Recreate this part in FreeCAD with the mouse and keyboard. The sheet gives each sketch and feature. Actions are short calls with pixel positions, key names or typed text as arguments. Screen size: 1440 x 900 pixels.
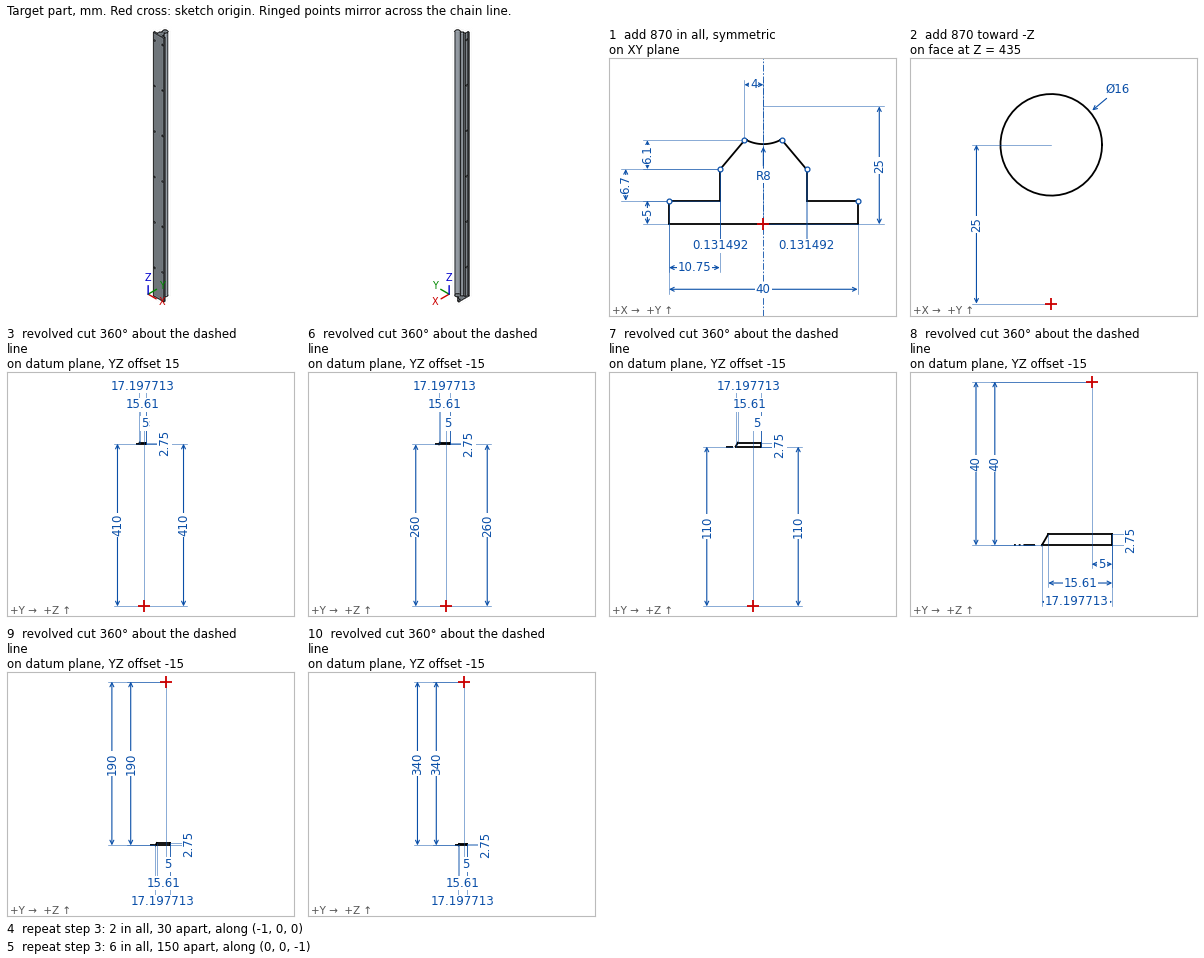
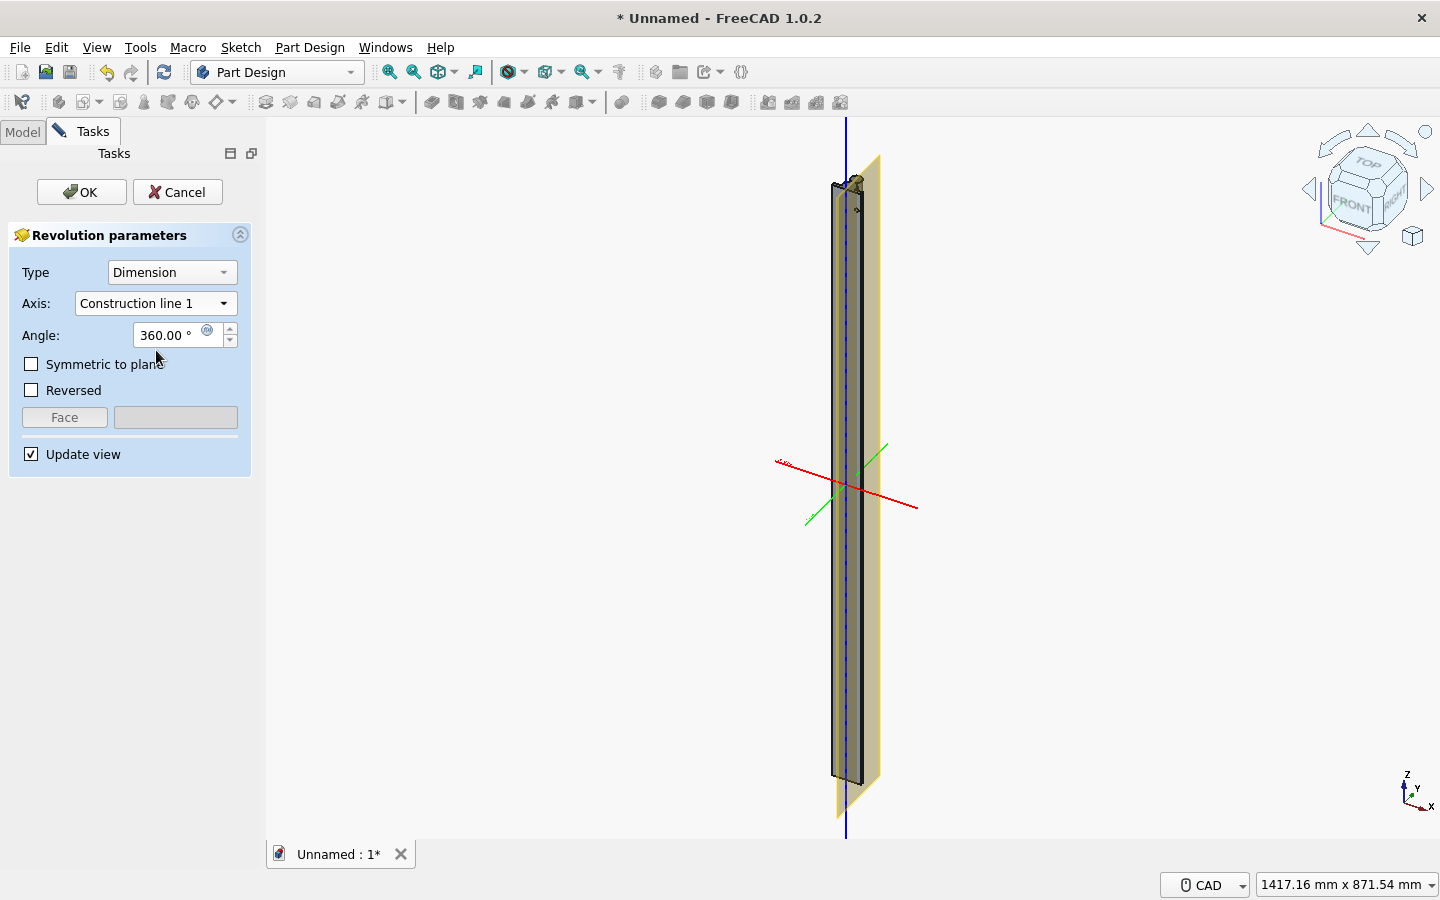
click(82, 192)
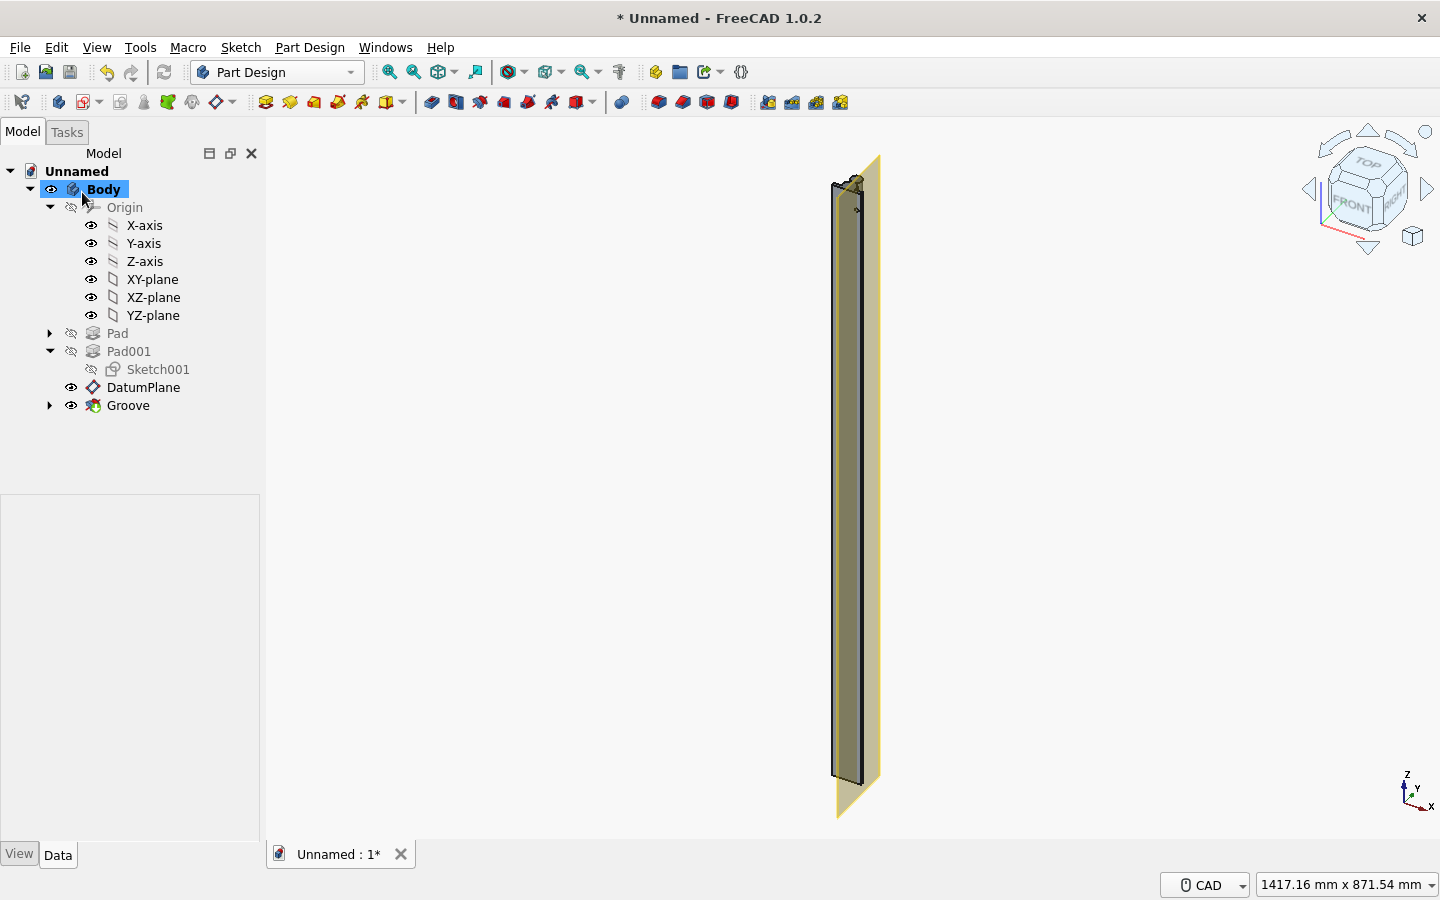
click(116, 387)
key(space)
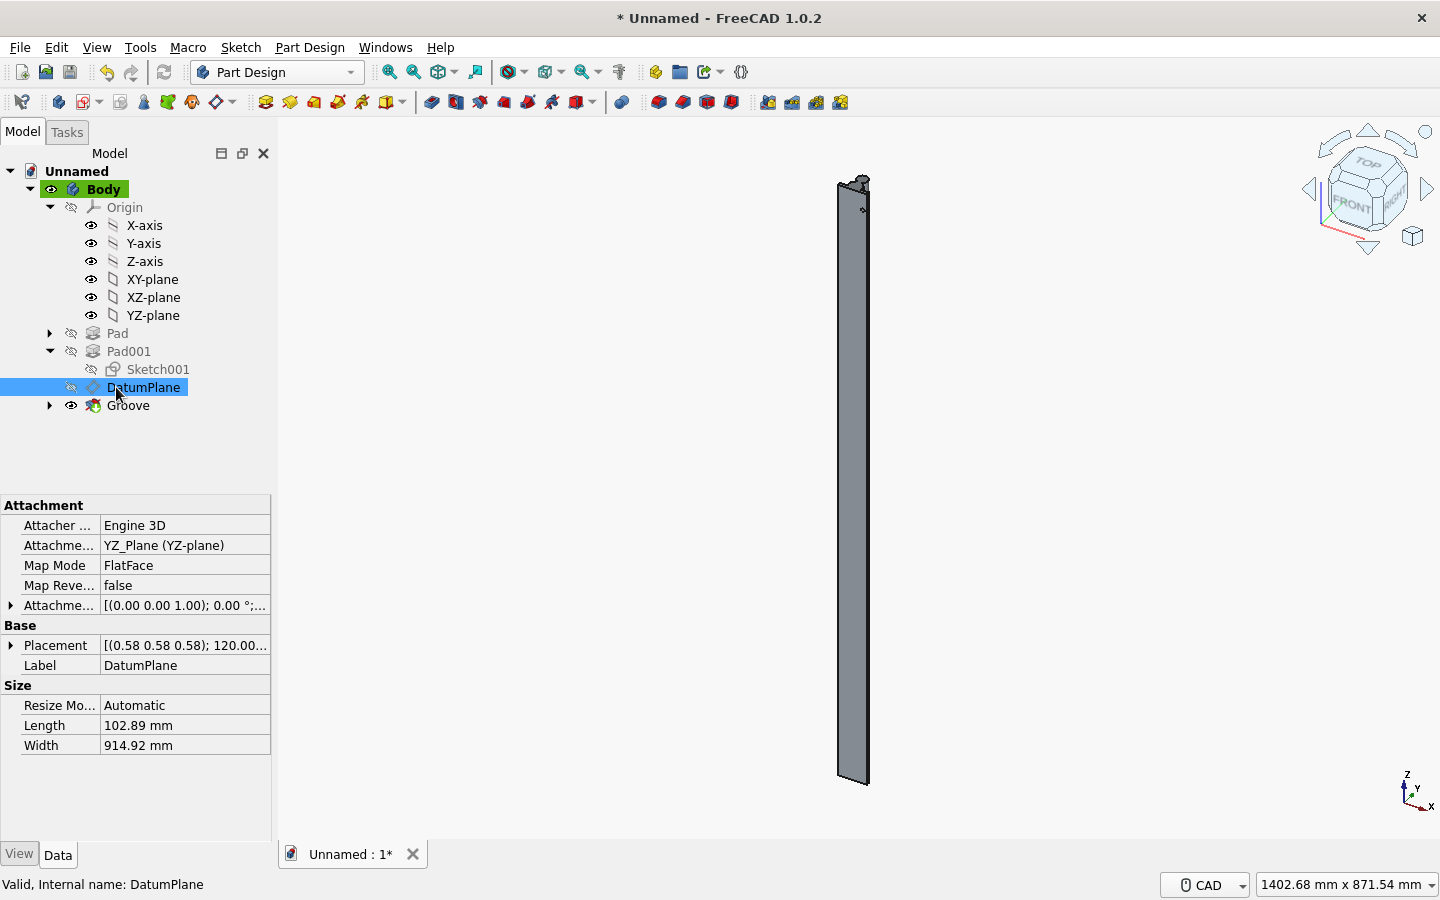
click(116, 405)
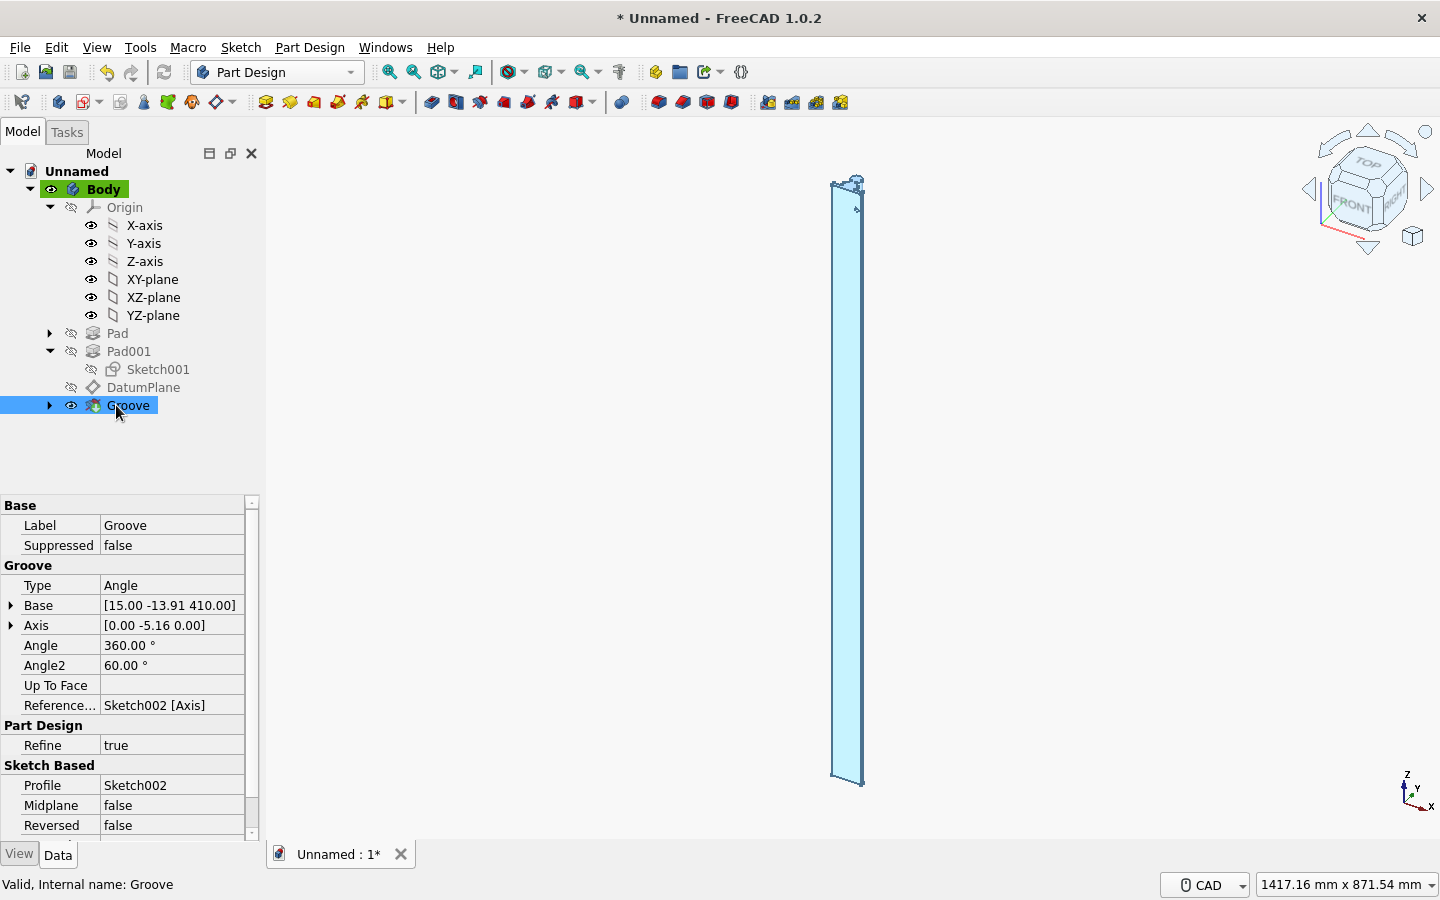
click(792, 102)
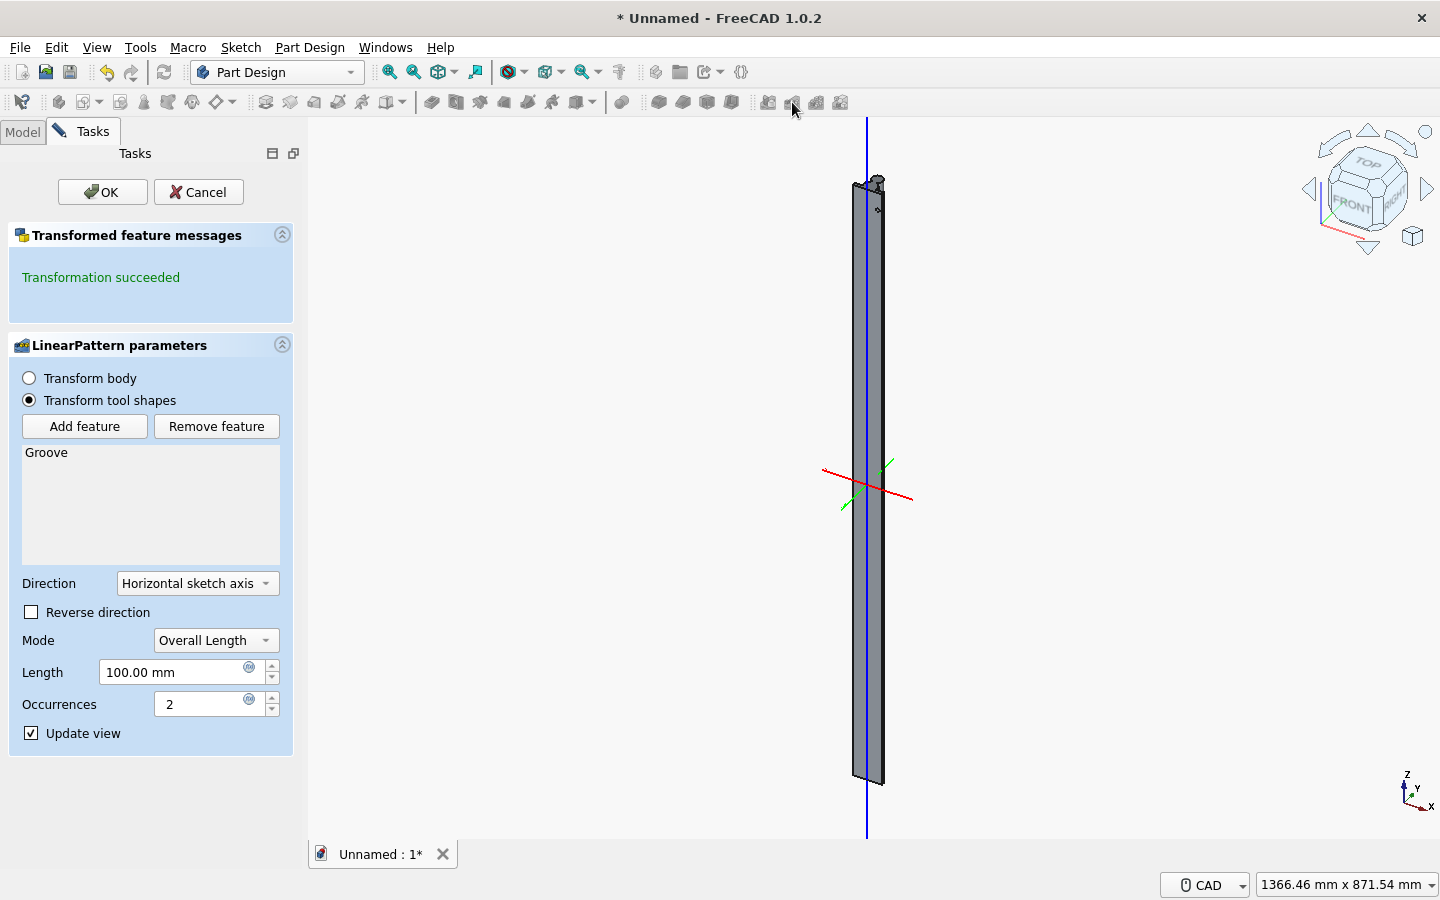
click(198, 584)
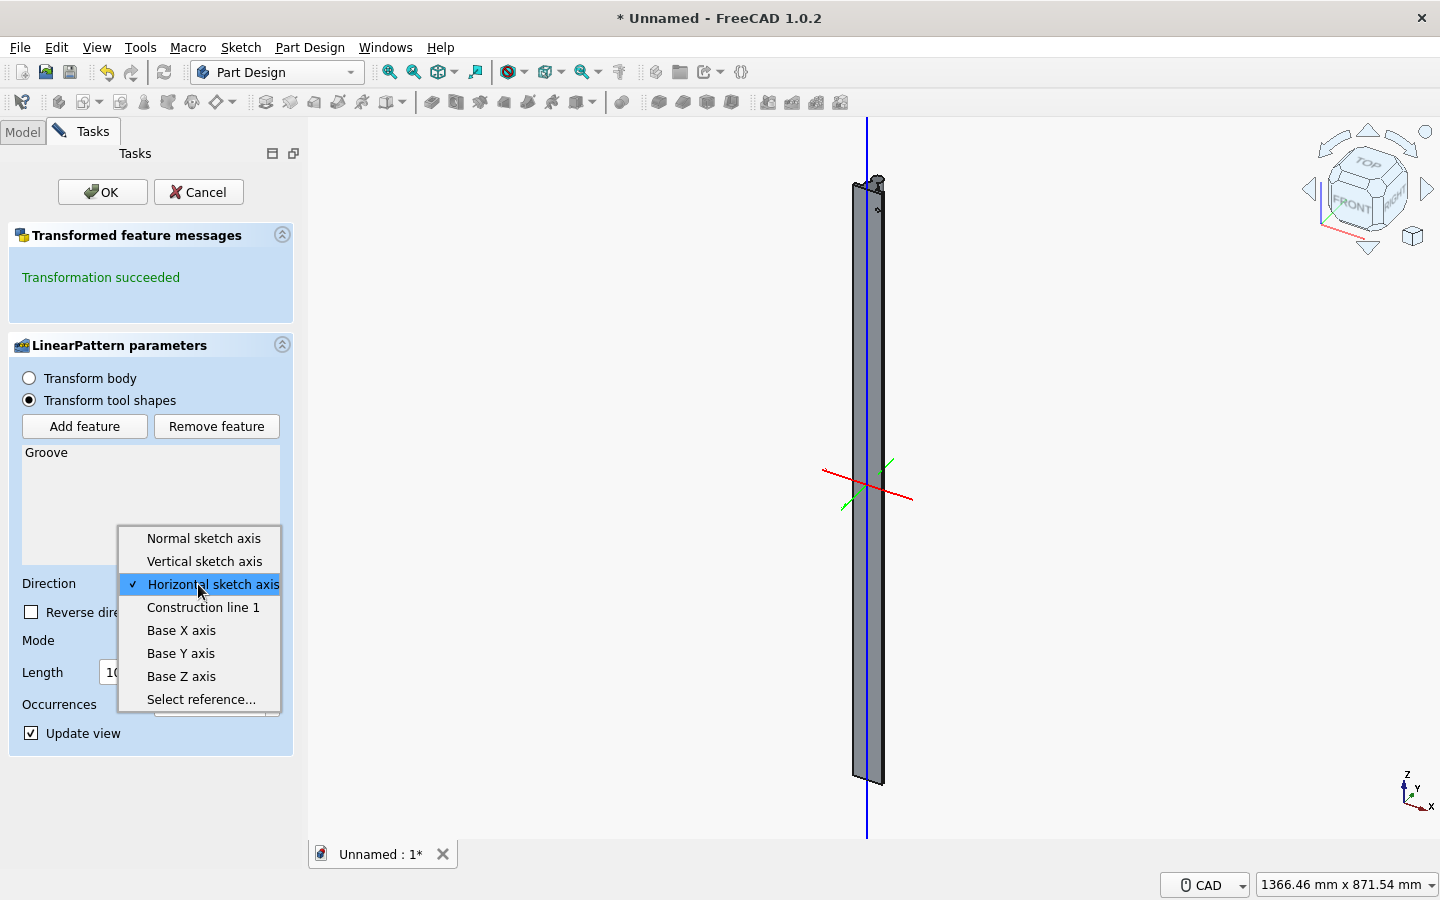
click(198, 630)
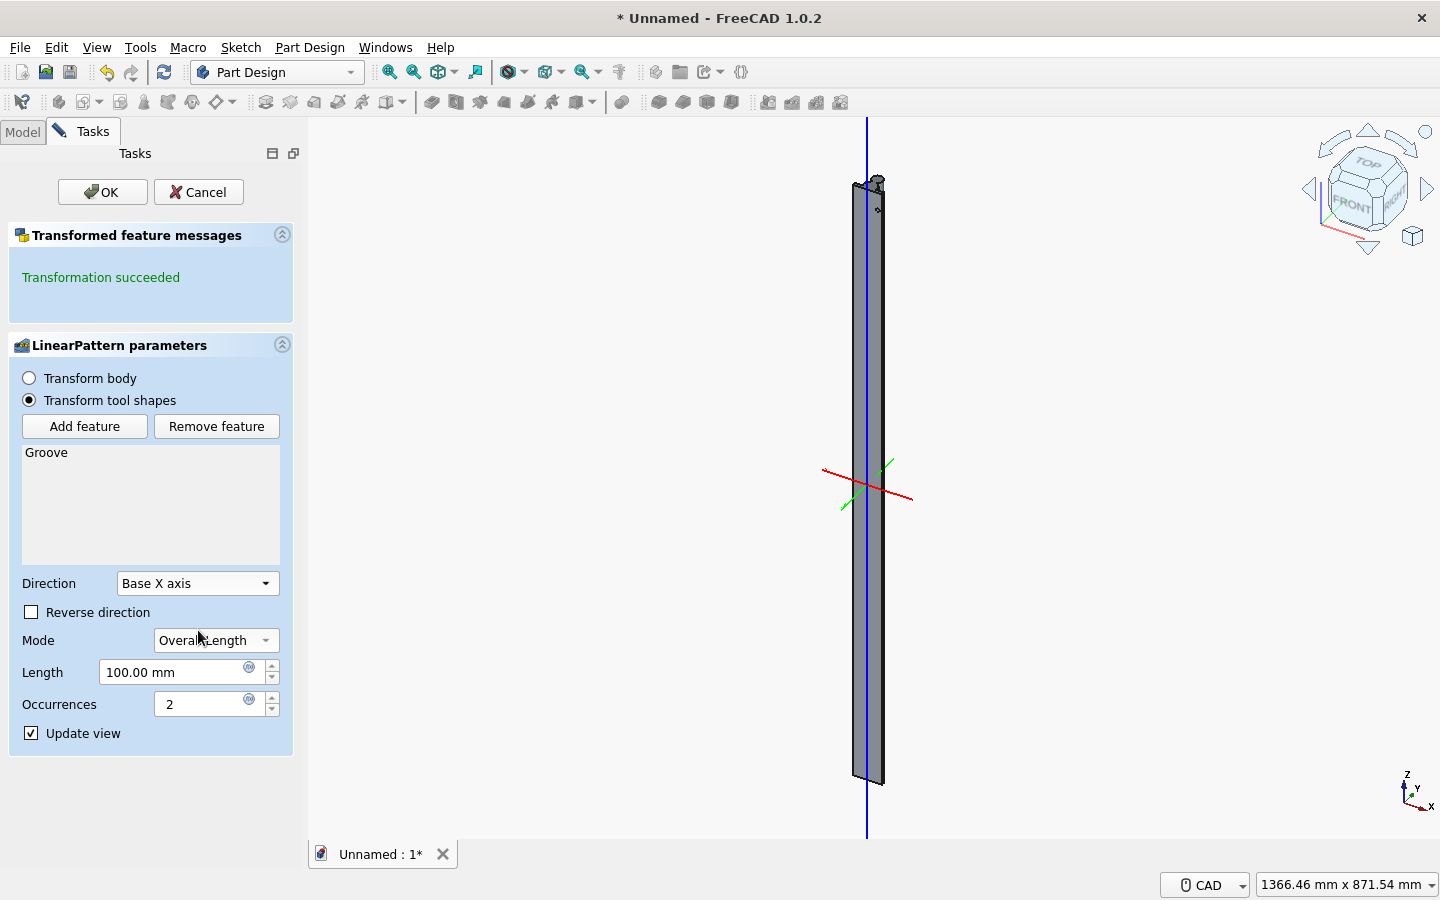
click(217, 640)